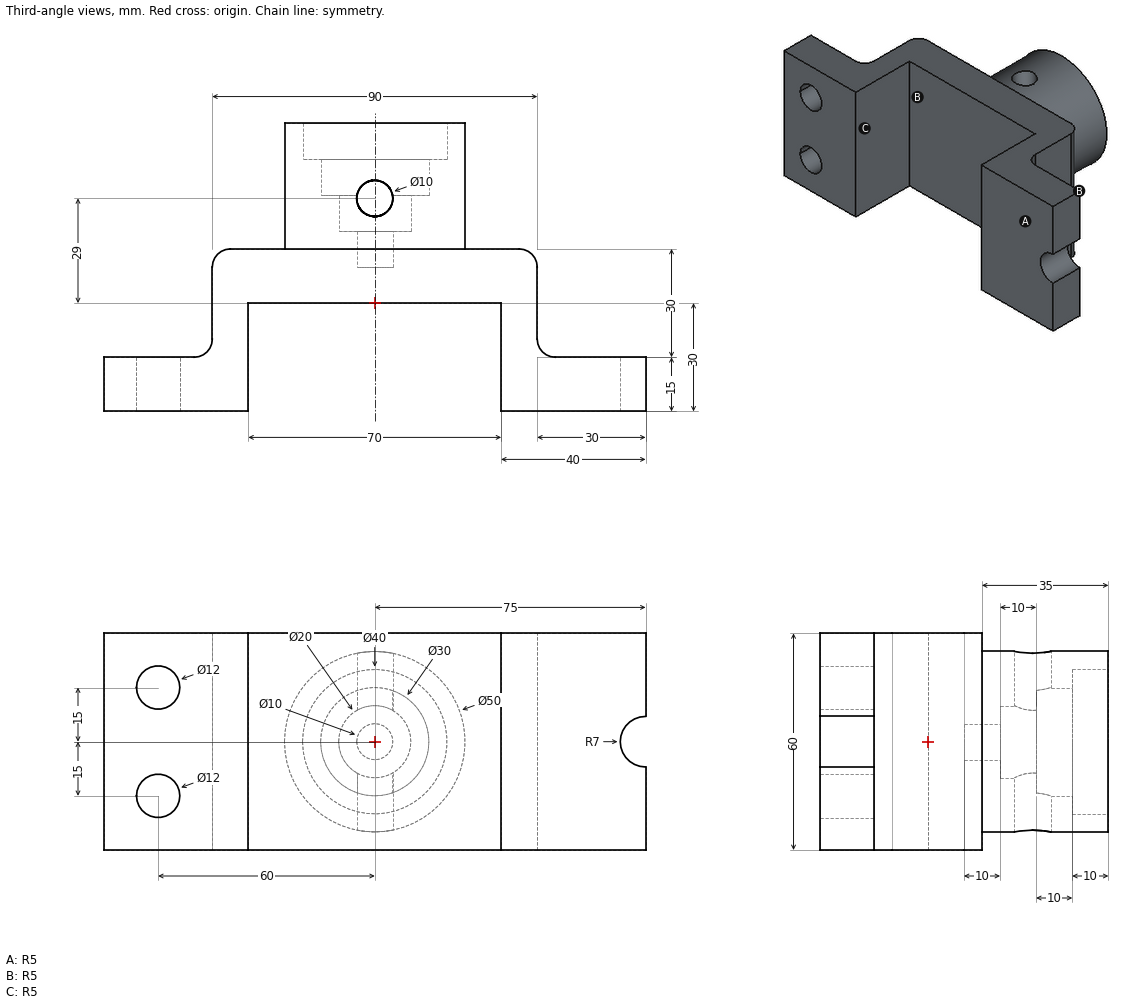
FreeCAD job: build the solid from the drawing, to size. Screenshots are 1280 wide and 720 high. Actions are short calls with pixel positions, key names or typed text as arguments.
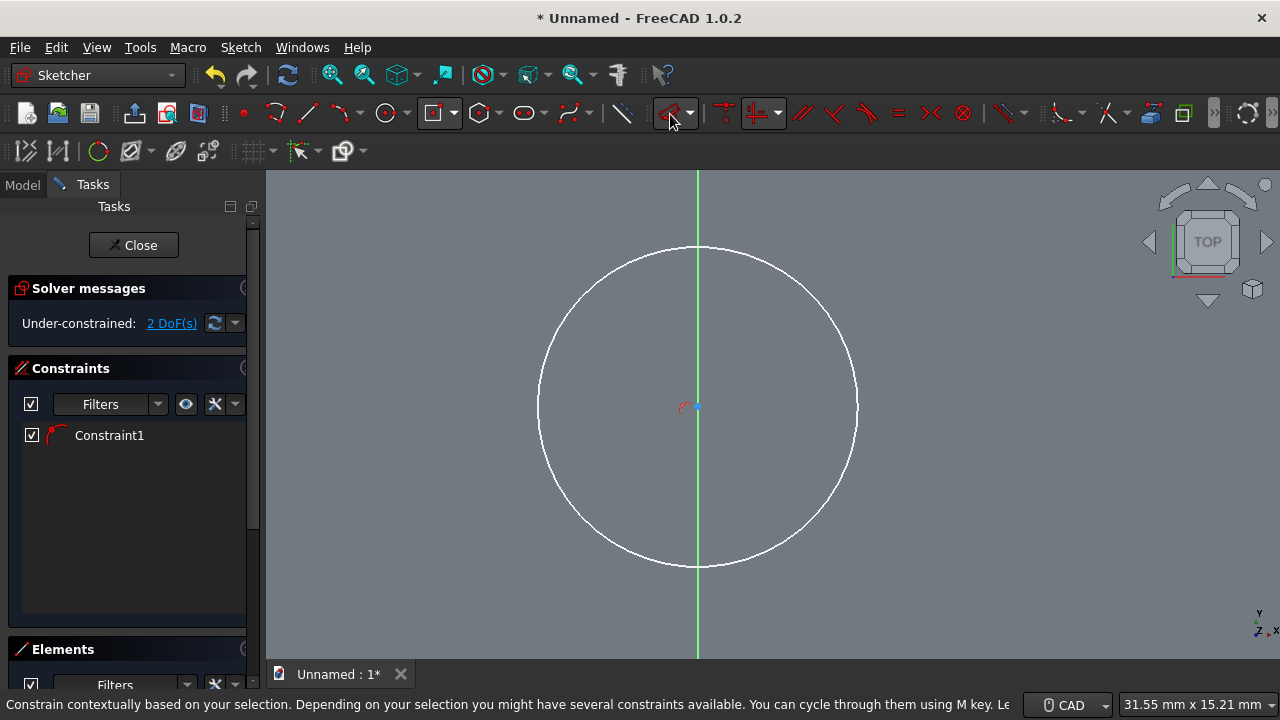
click(811, 294)
click(834, 271)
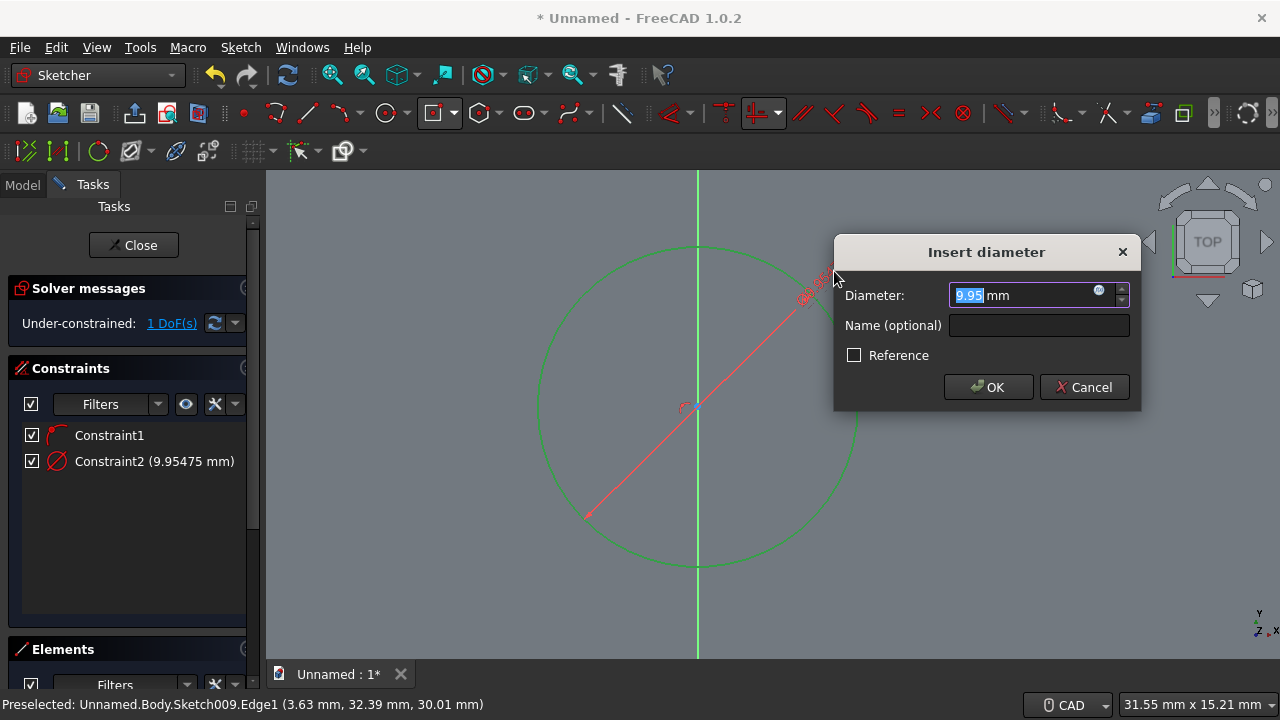
text(10)
key(Return)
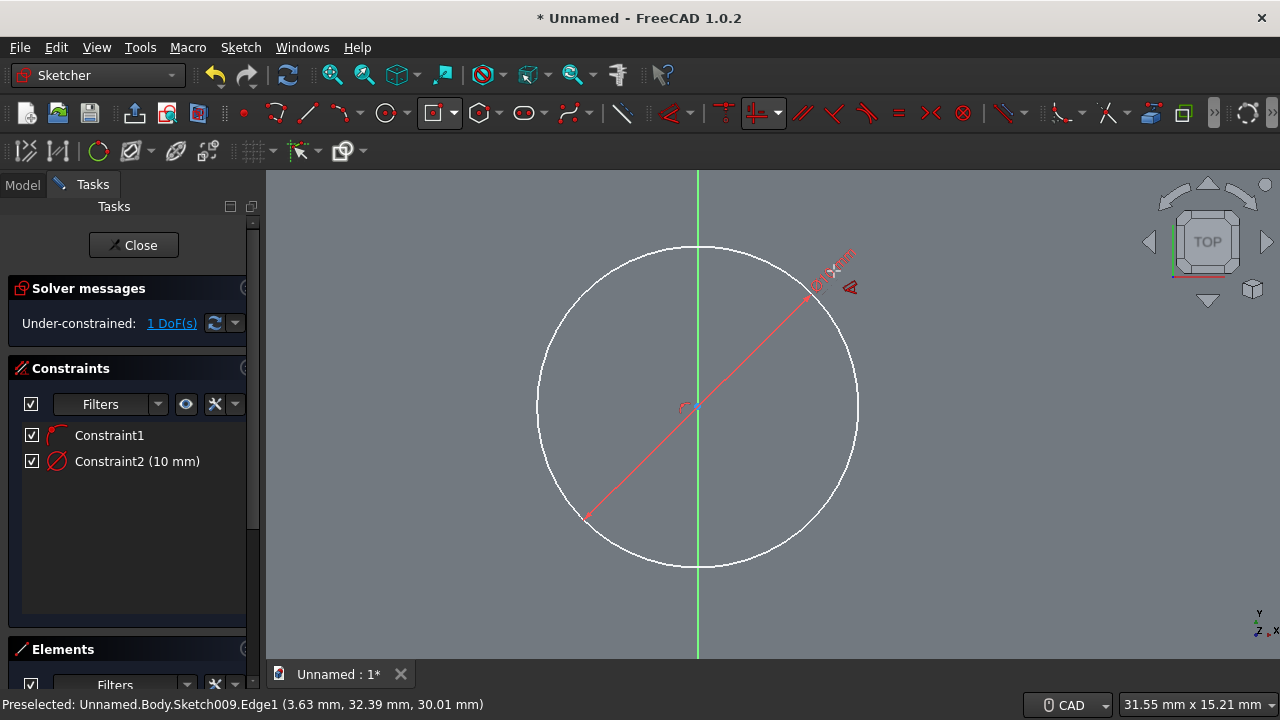
click(698, 407)
click(732, 519)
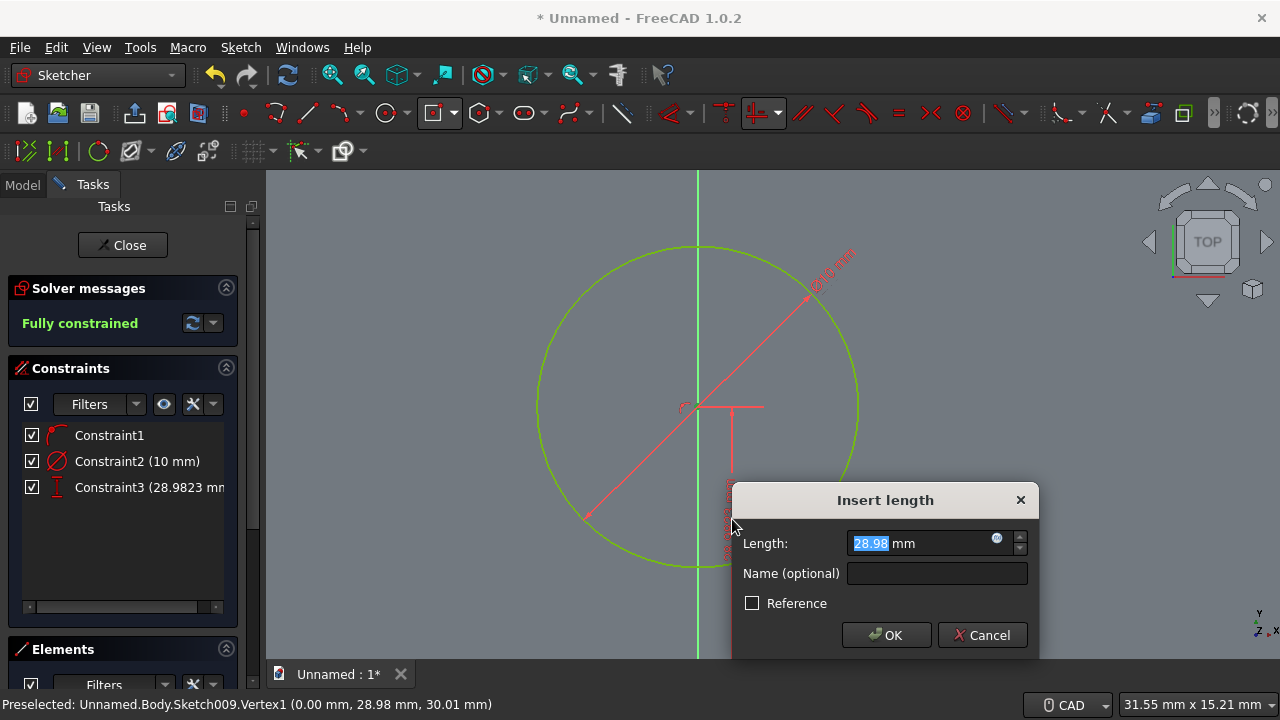
text(29)
key(Return)
key(Escape)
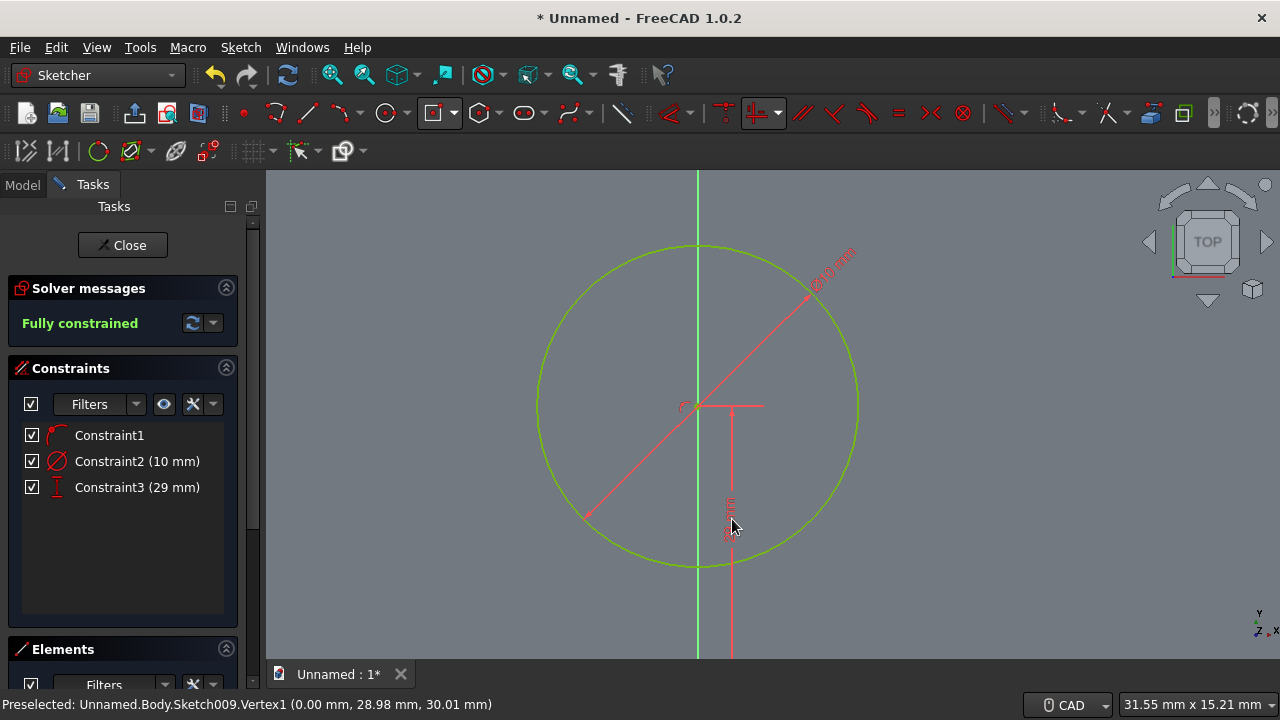
click(123, 245)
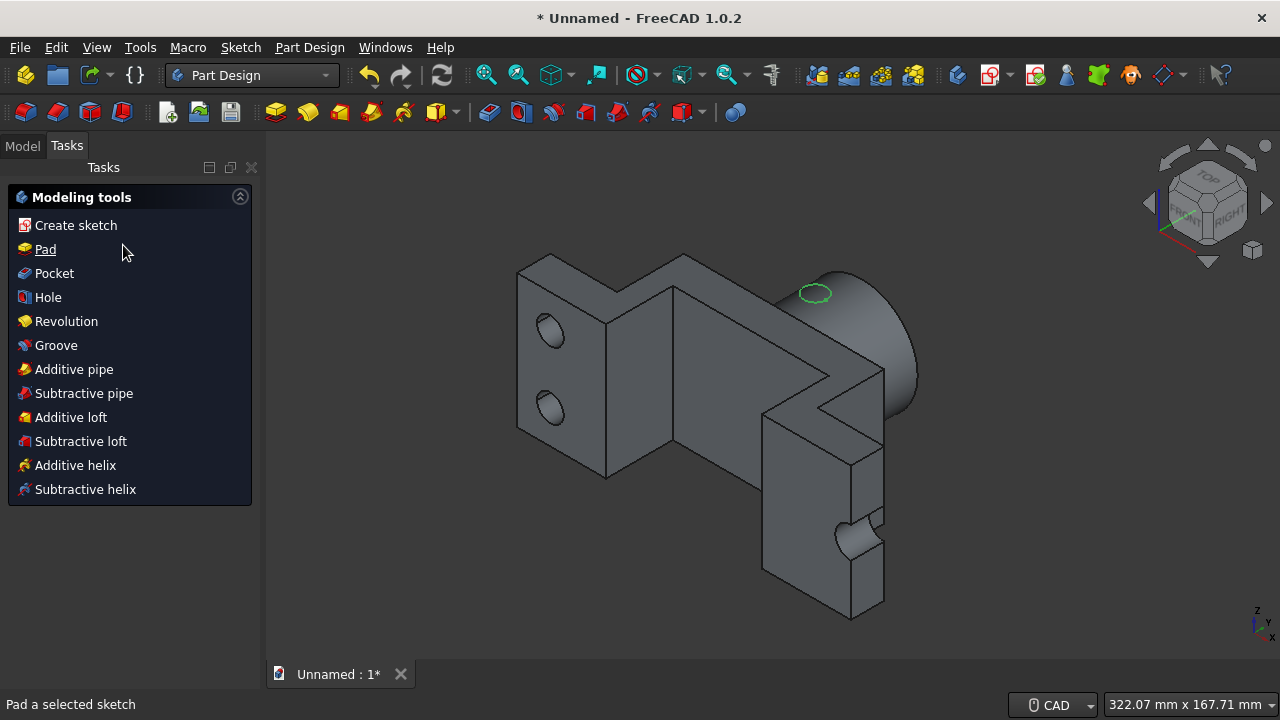
click(490, 112)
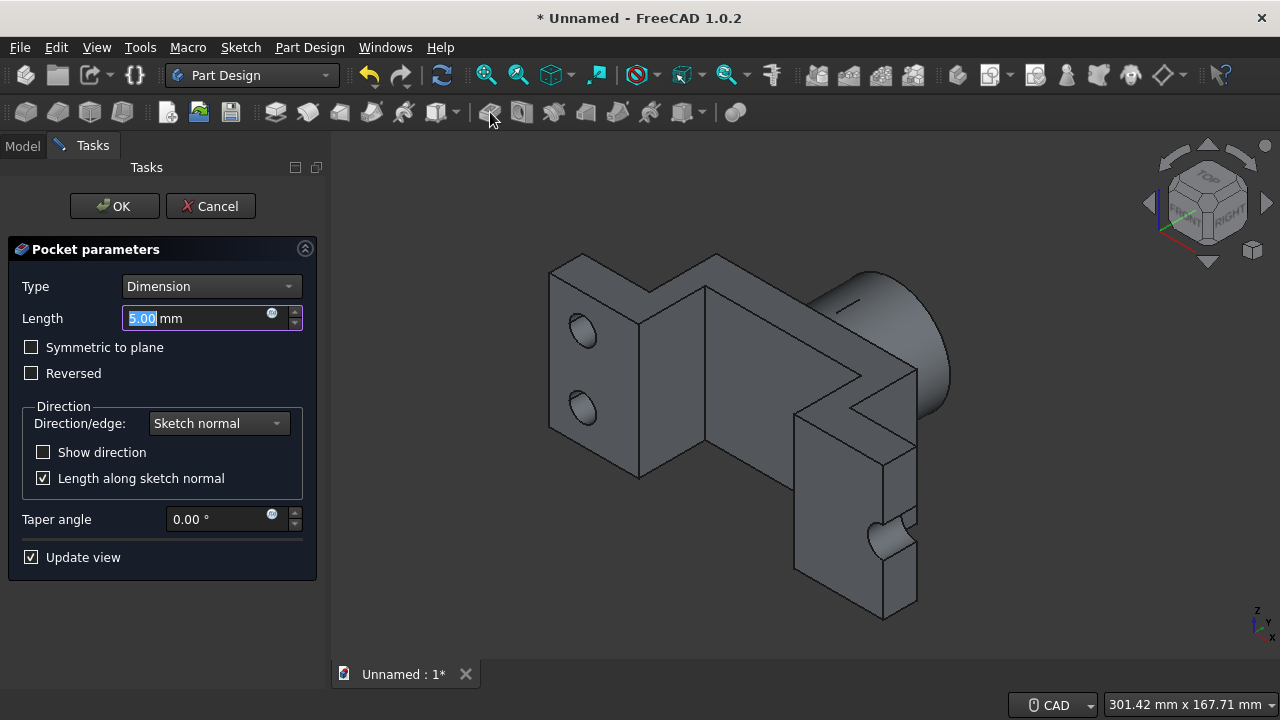
click(212, 286)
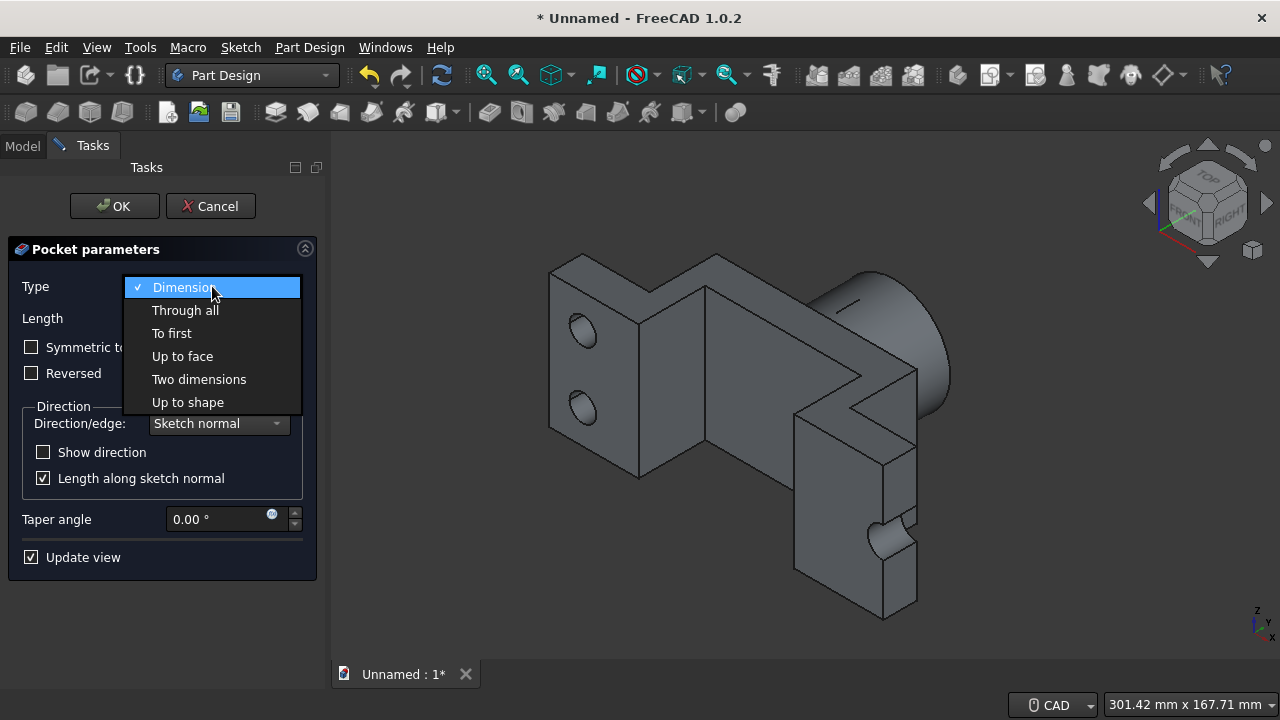
click(212, 310)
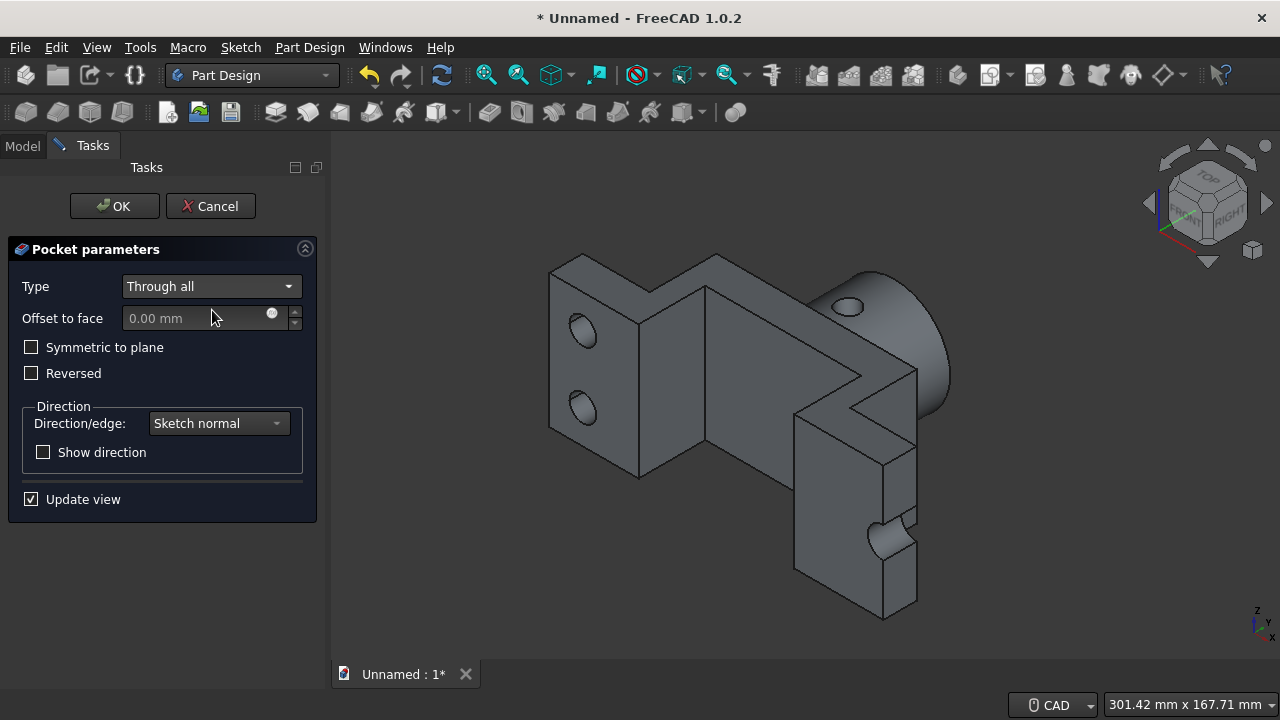
click(115, 206)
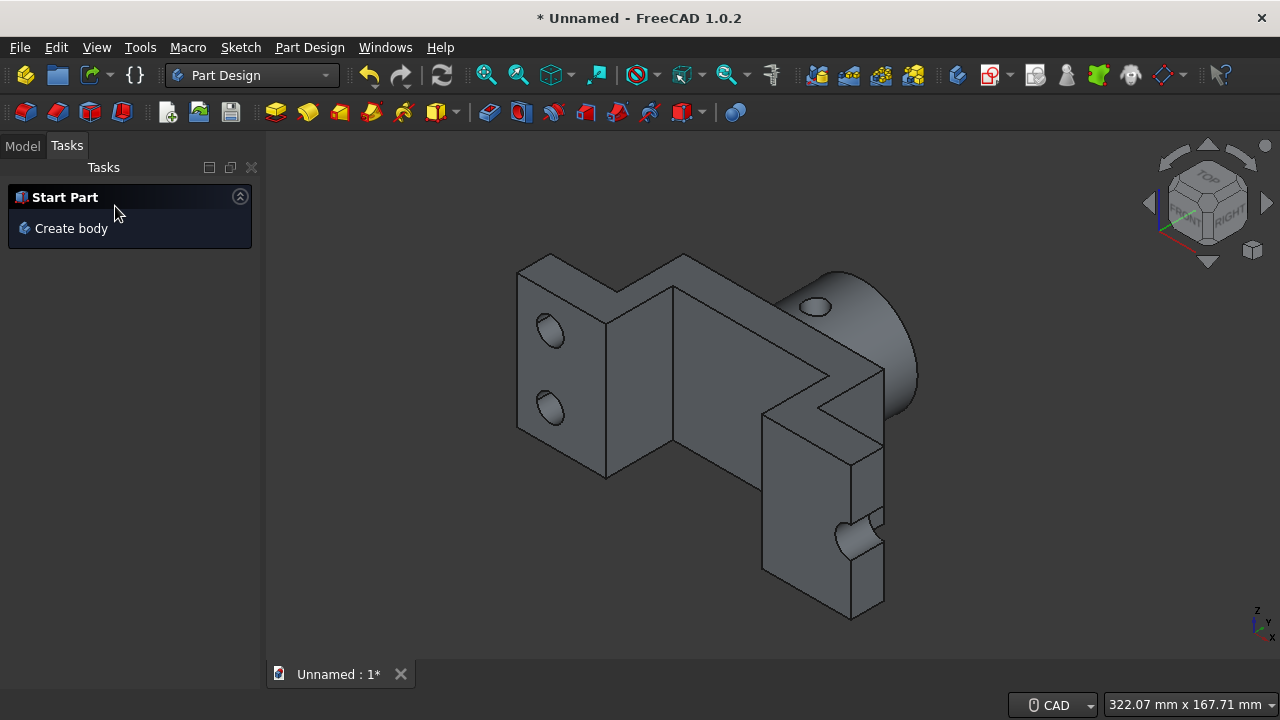
key(2)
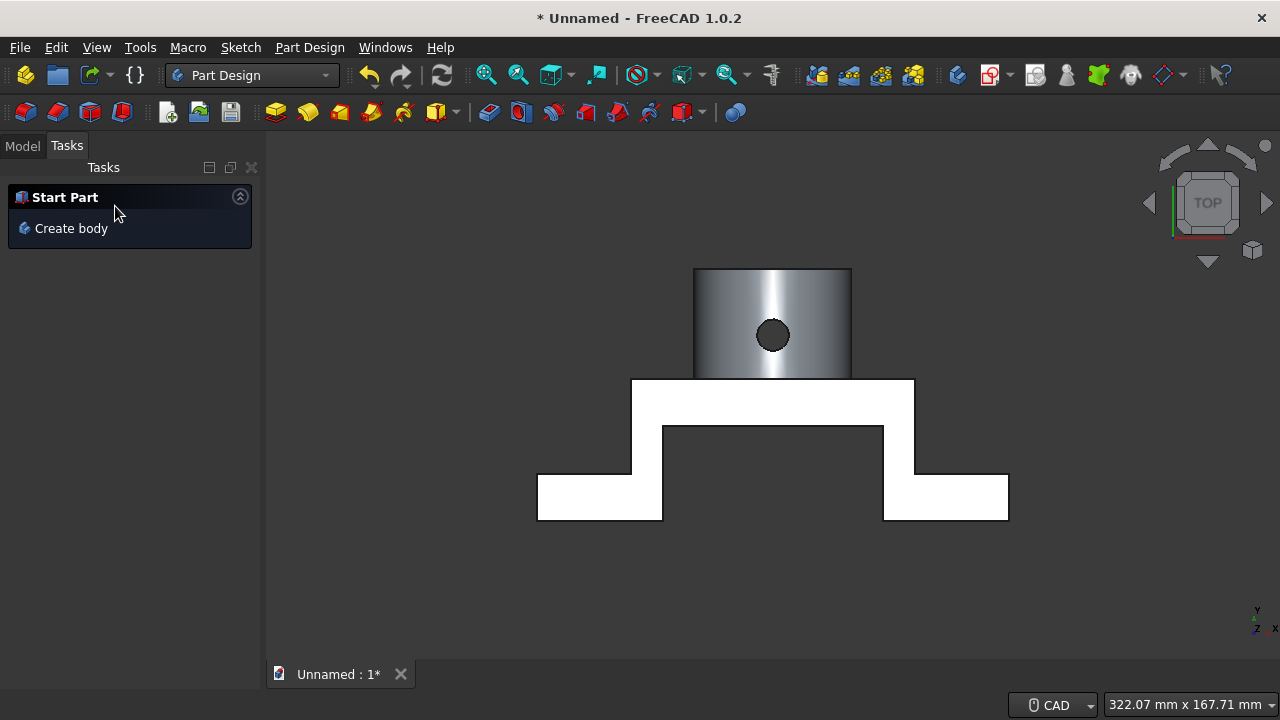
key(0)